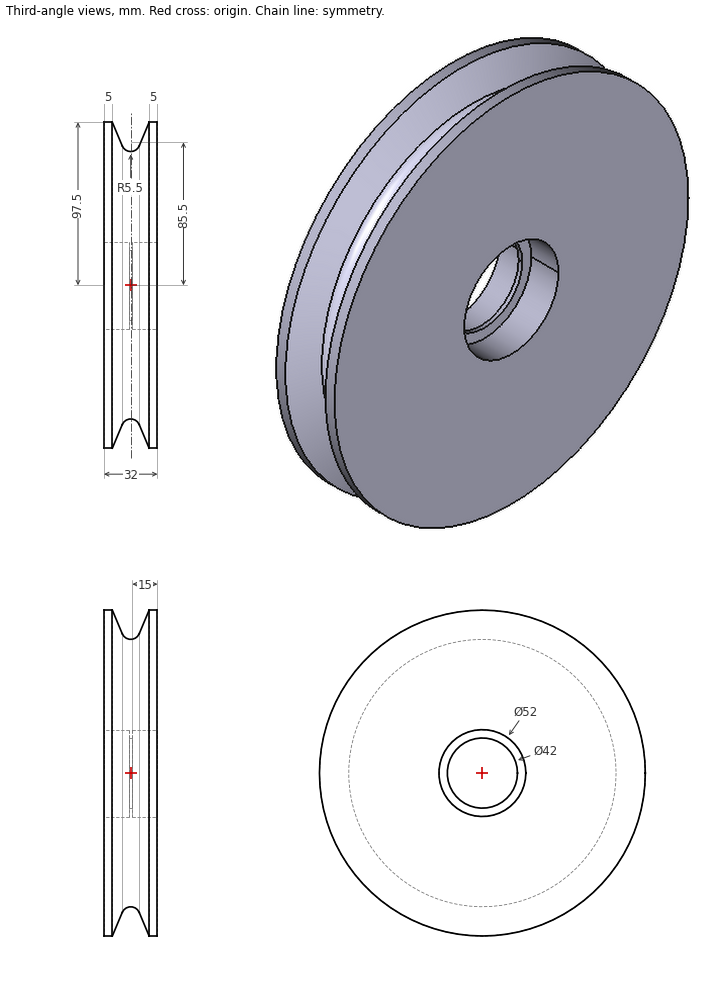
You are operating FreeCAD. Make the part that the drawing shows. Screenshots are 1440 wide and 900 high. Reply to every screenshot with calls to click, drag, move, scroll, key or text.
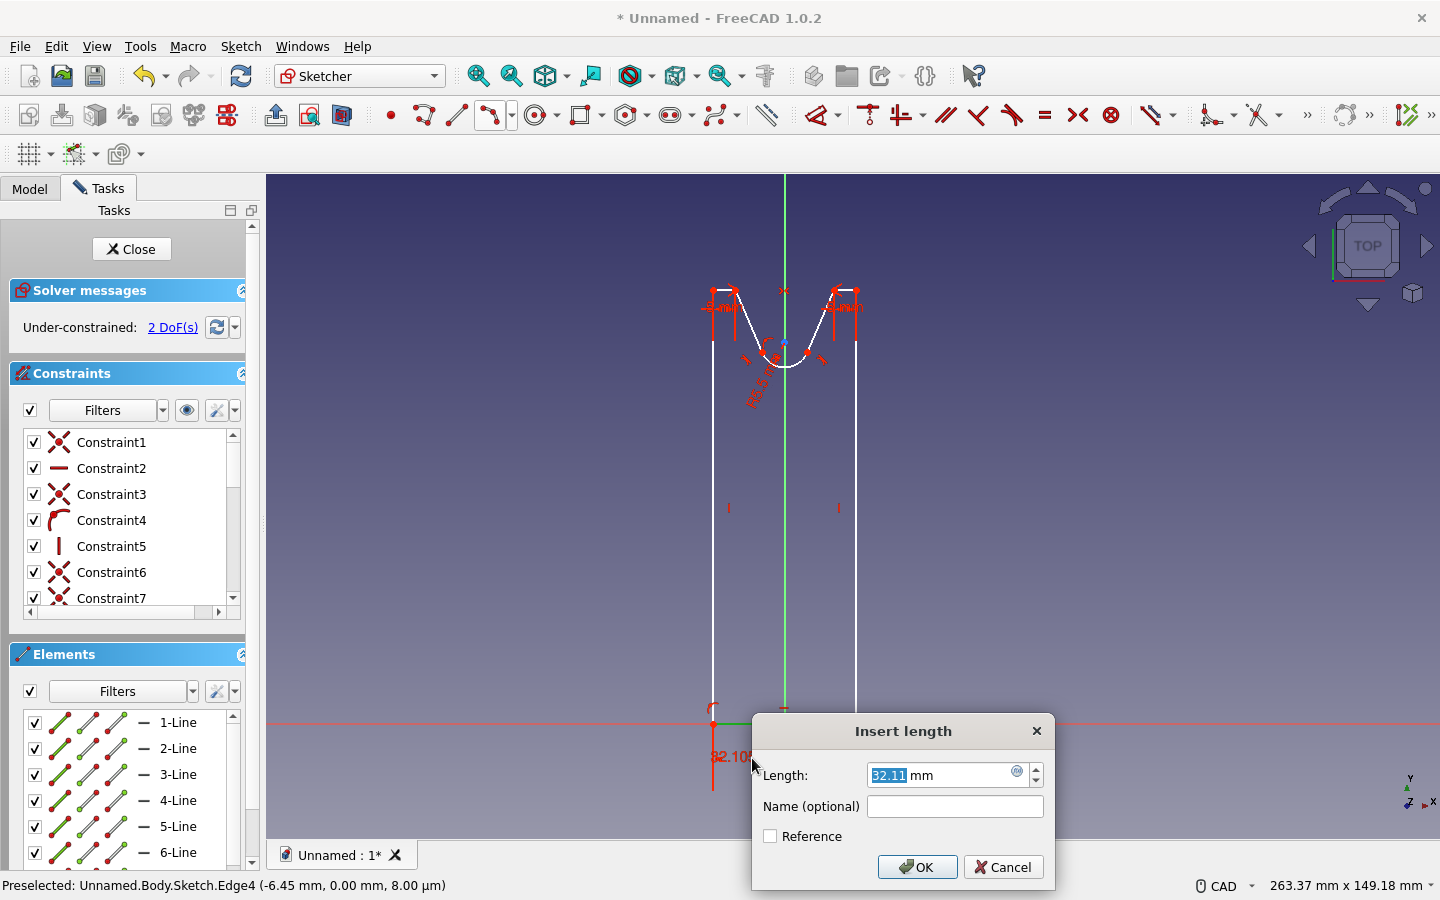
text(32)
key(Return)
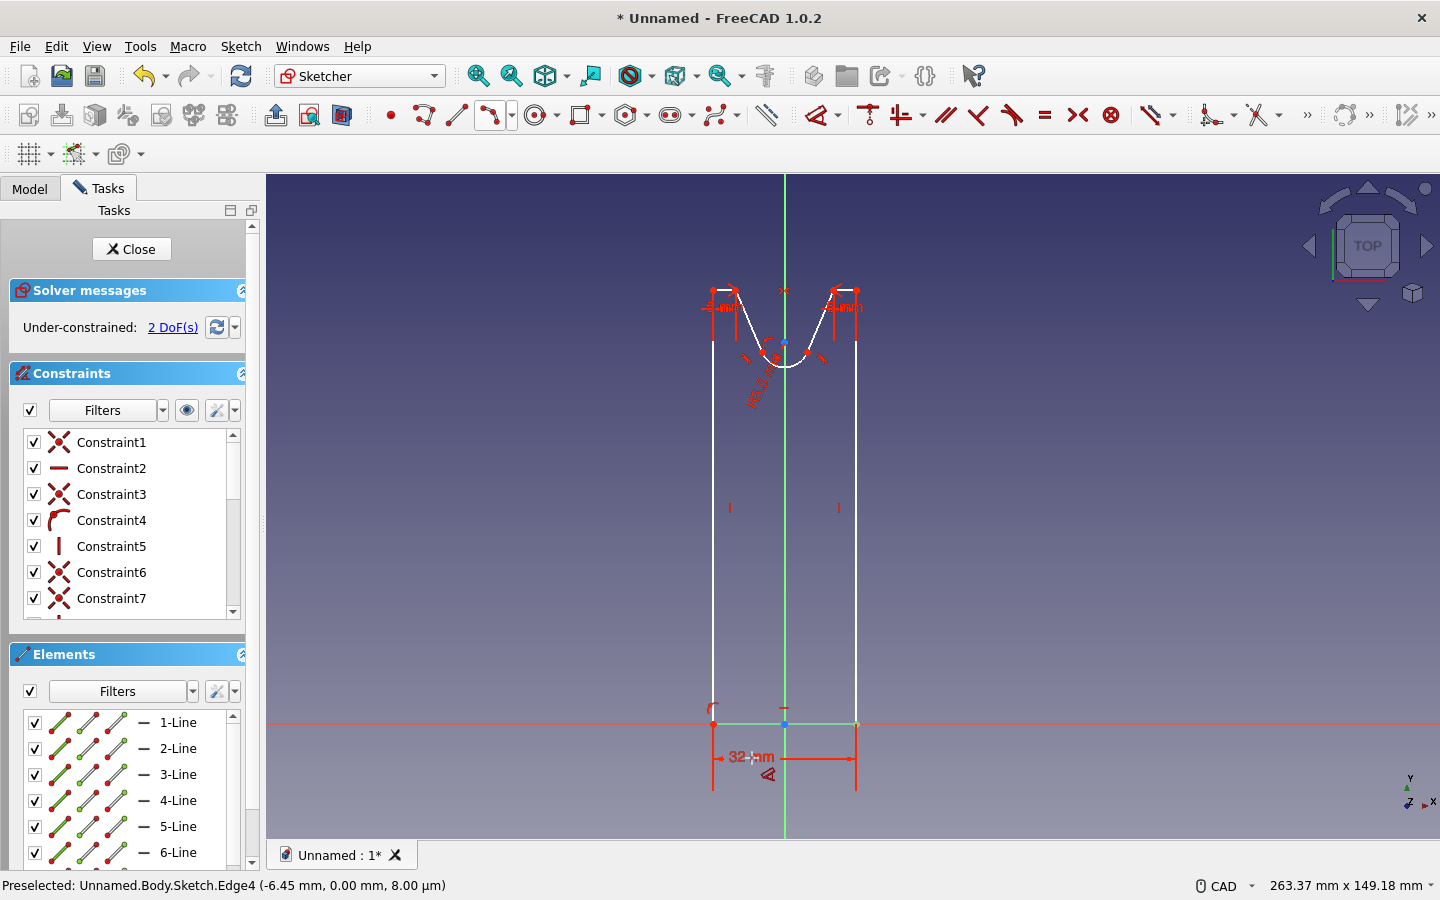
click(713, 420)
click(679, 507)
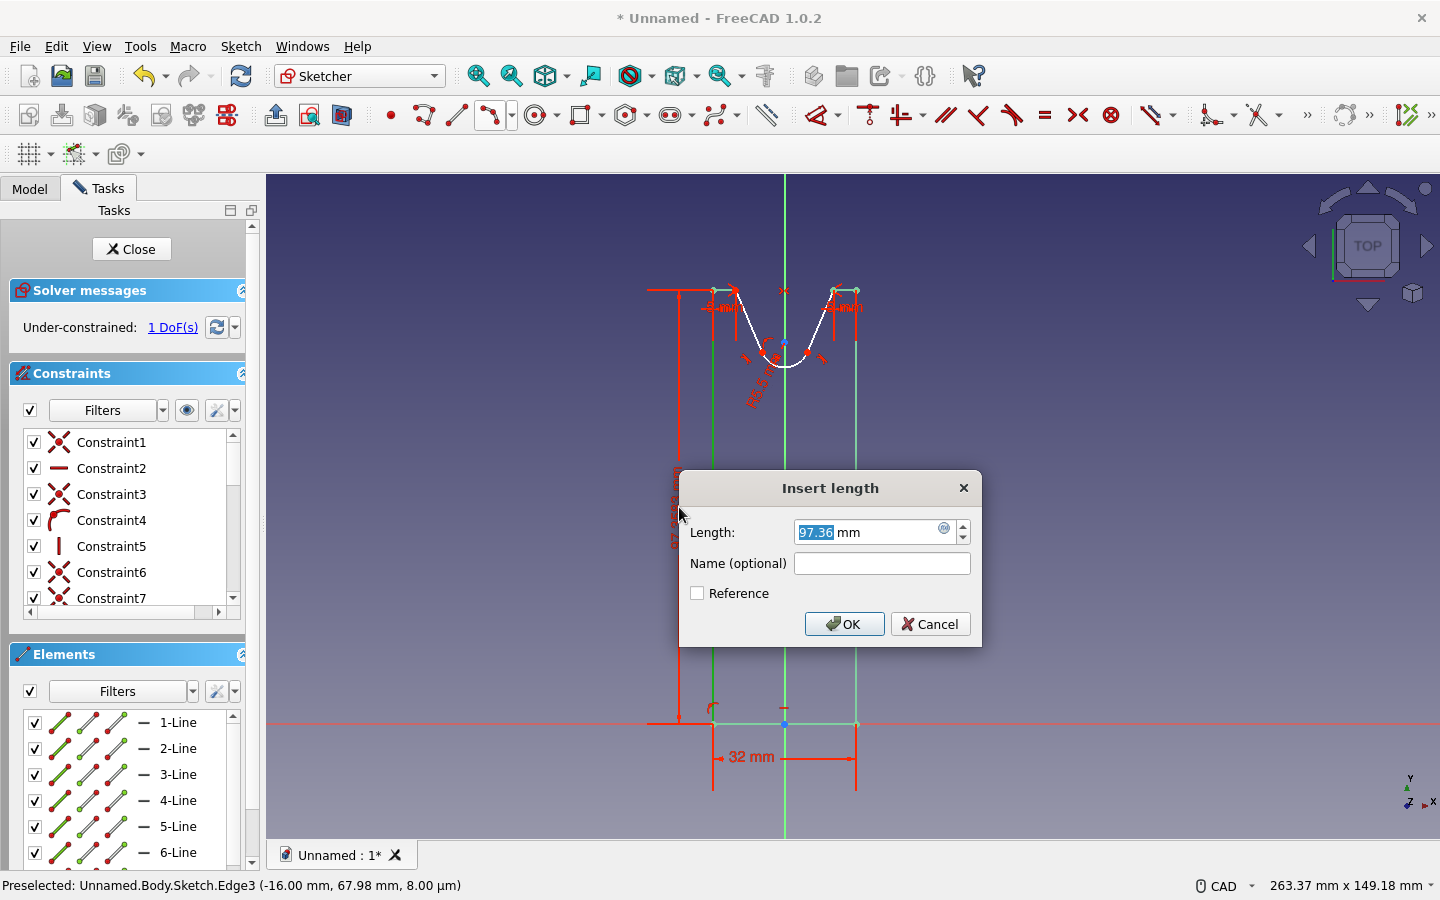
text(97.5)
key(Return)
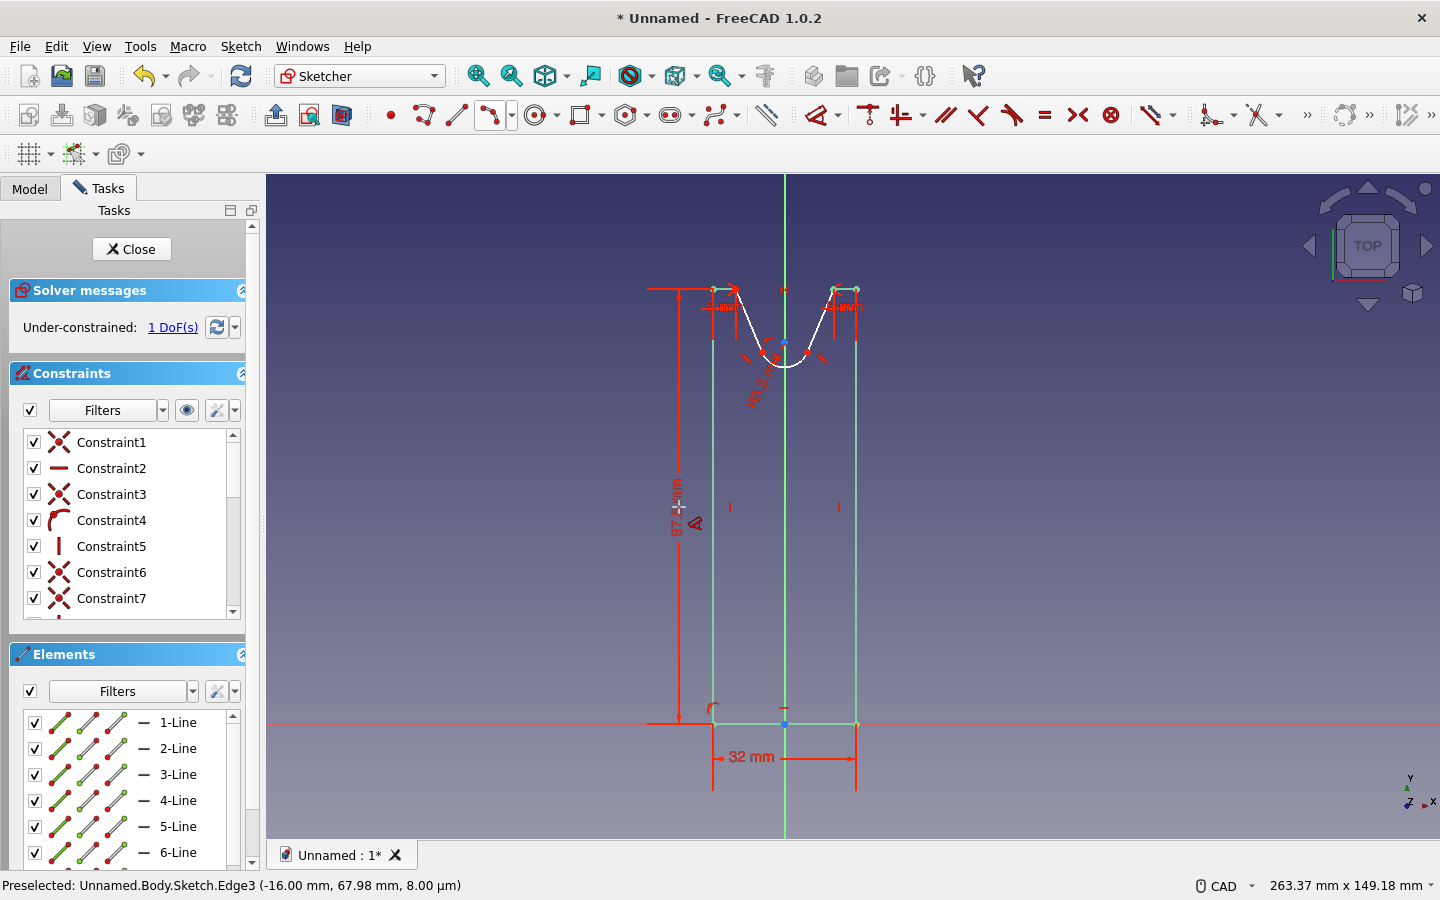
click(785, 343)
click(819, 533)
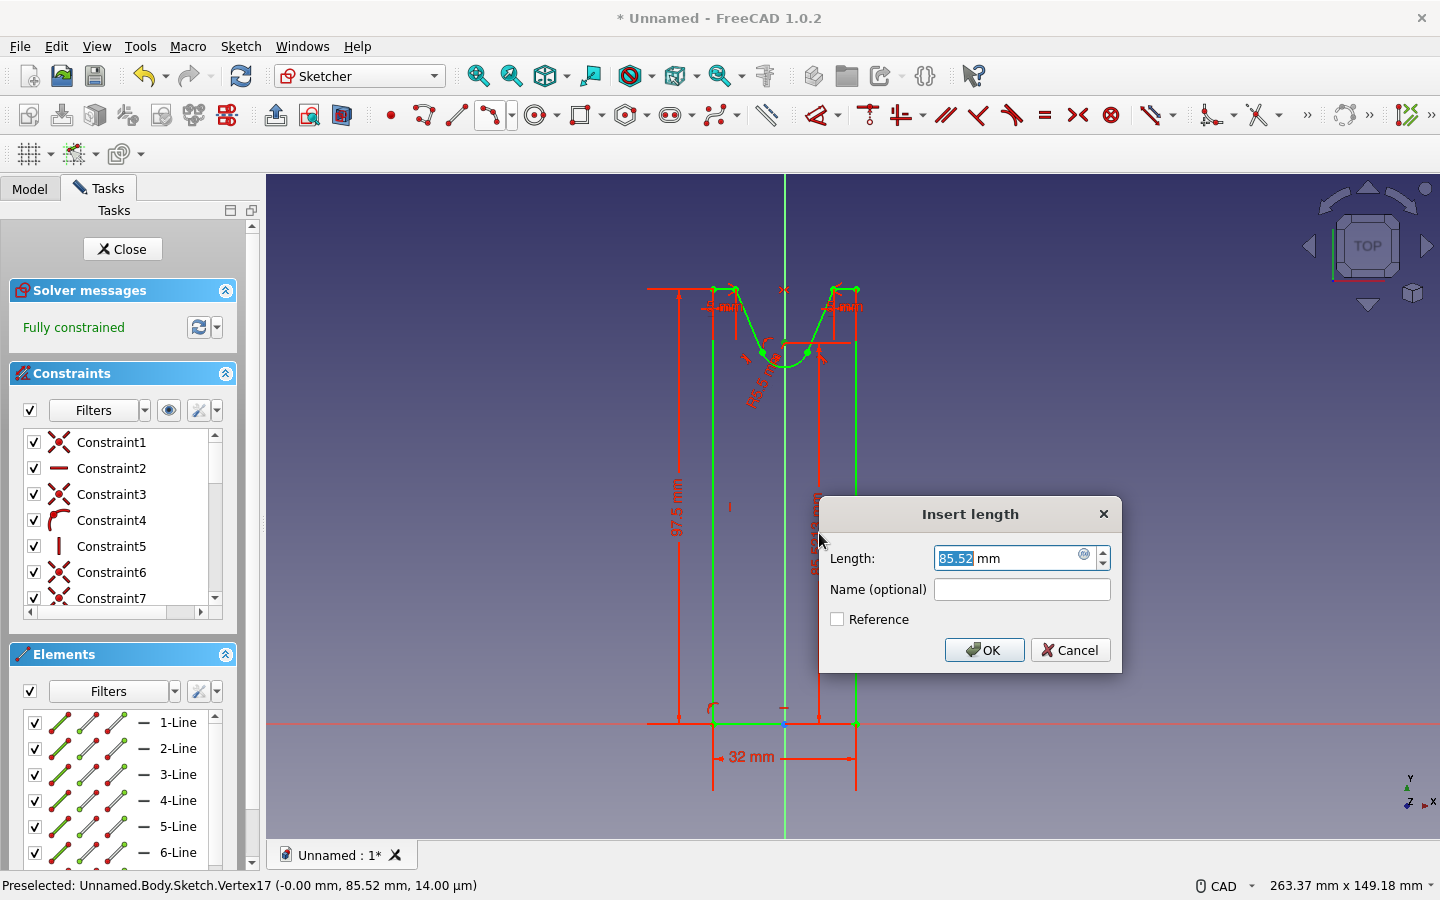
text(85.5)
key(Return)
key(Escape)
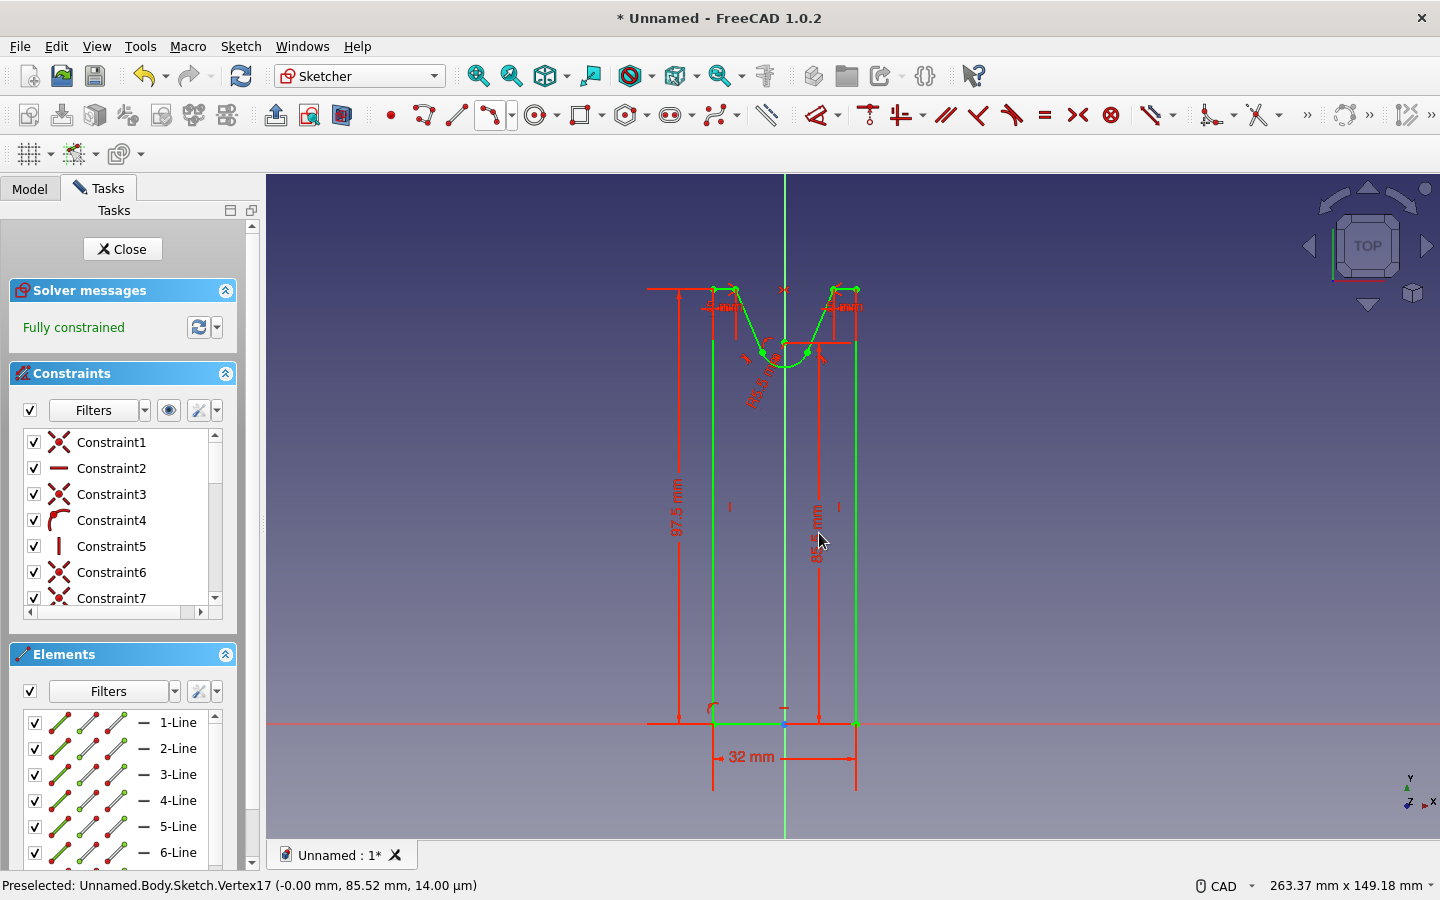
click(123, 249)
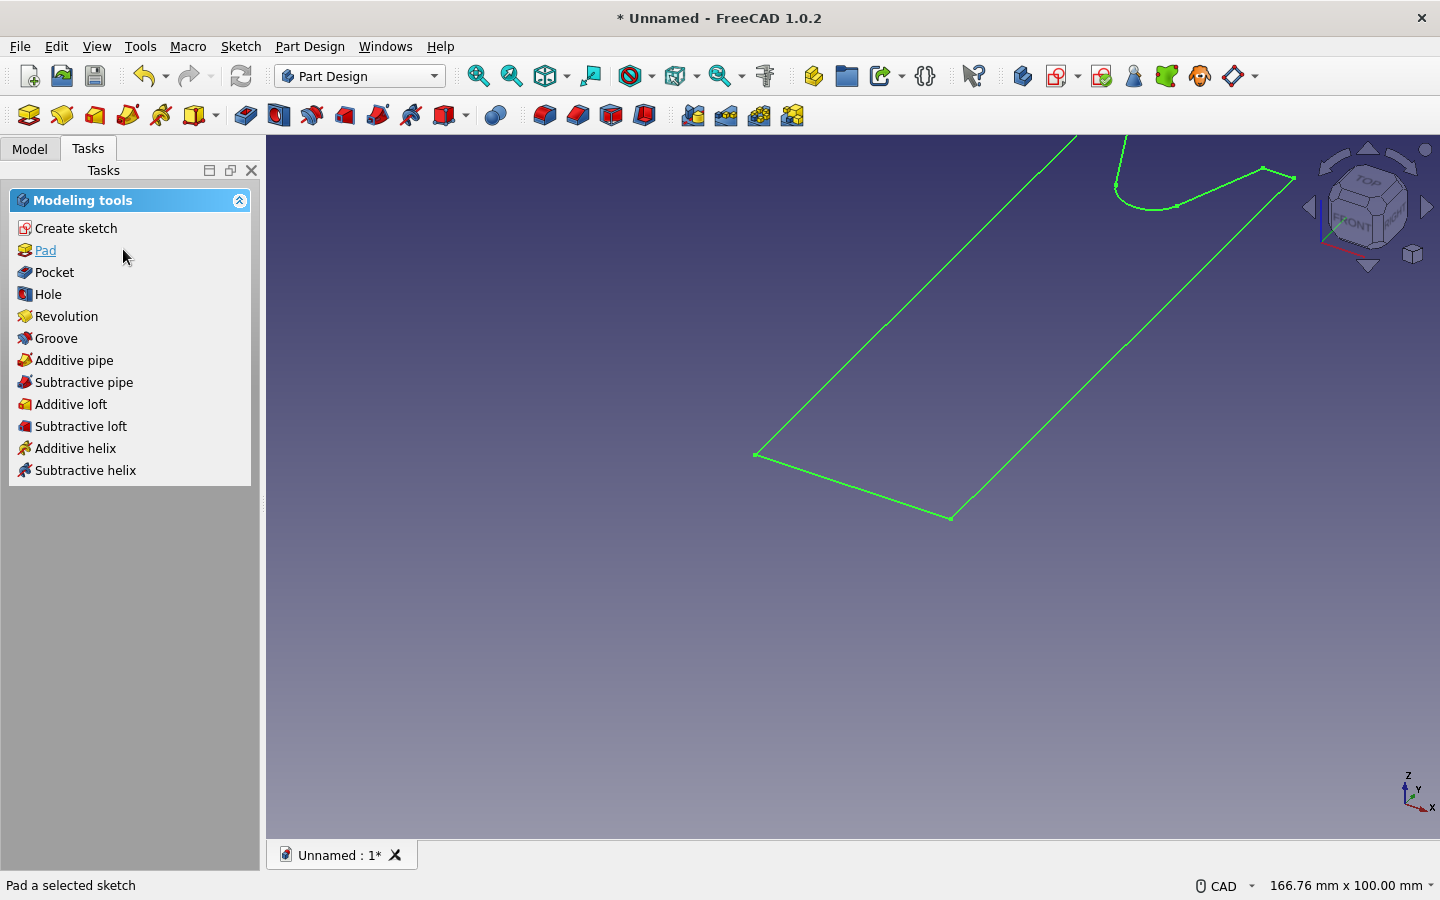
click(62, 116)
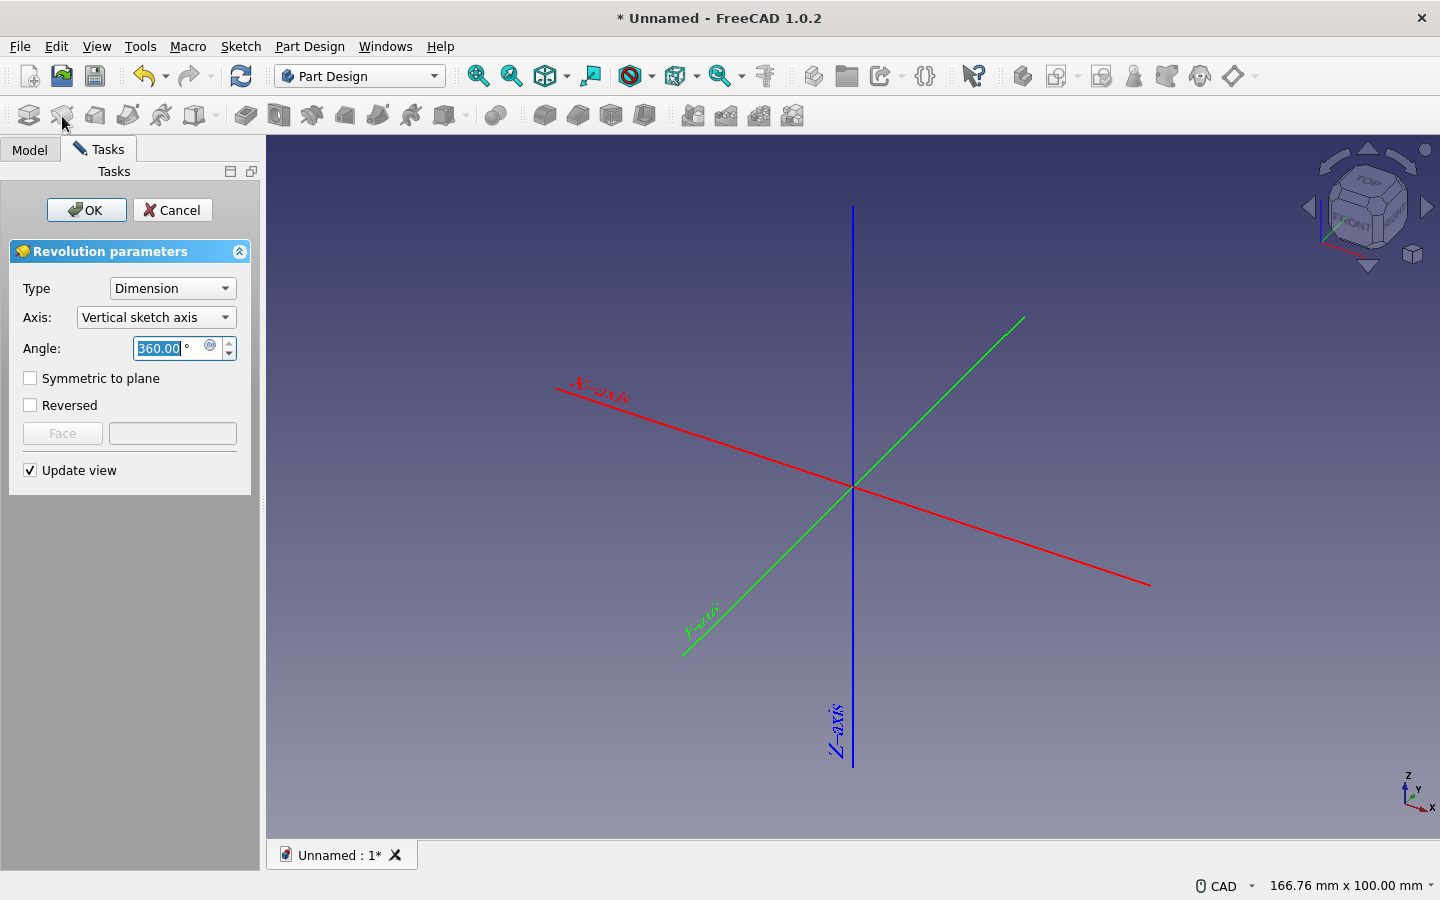
click(157, 318)